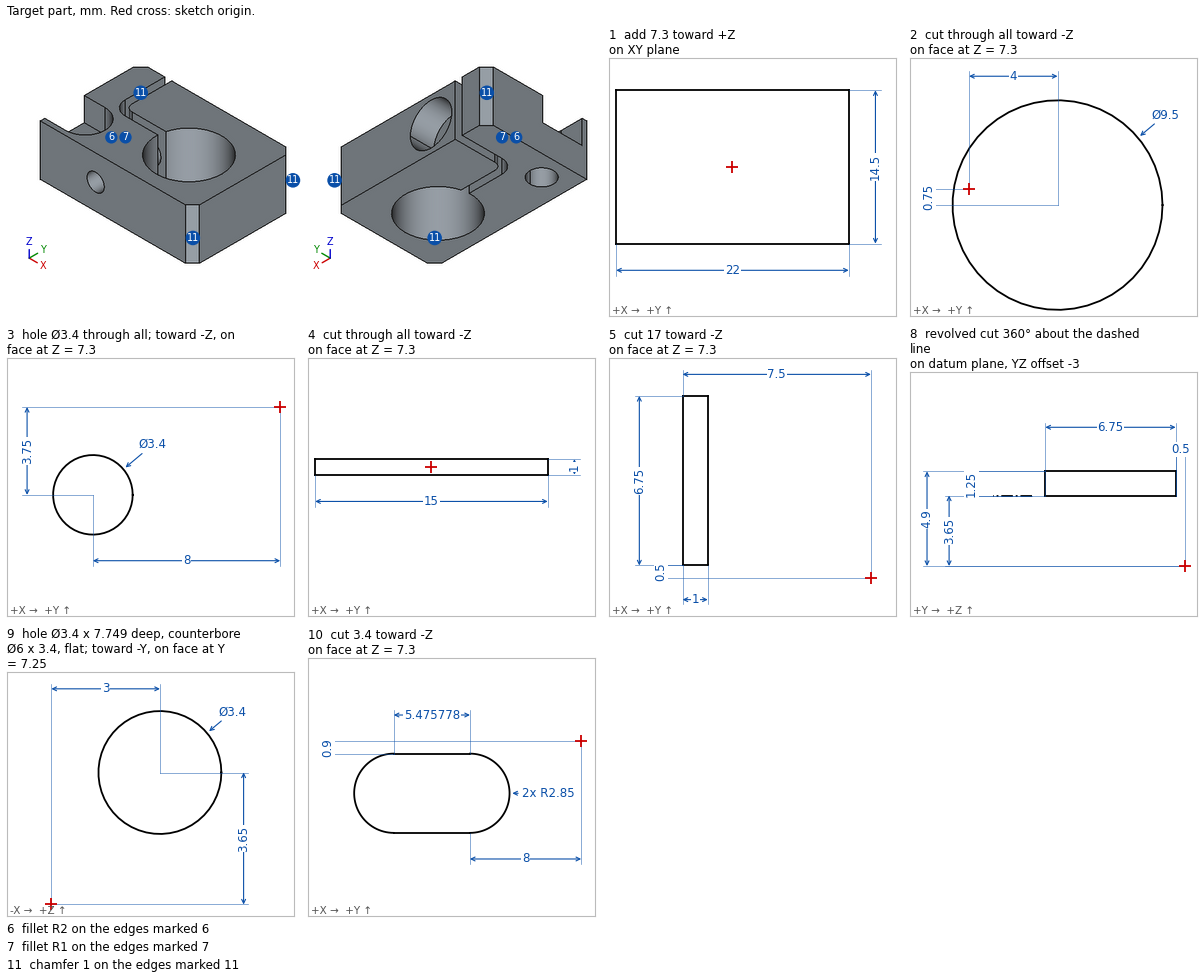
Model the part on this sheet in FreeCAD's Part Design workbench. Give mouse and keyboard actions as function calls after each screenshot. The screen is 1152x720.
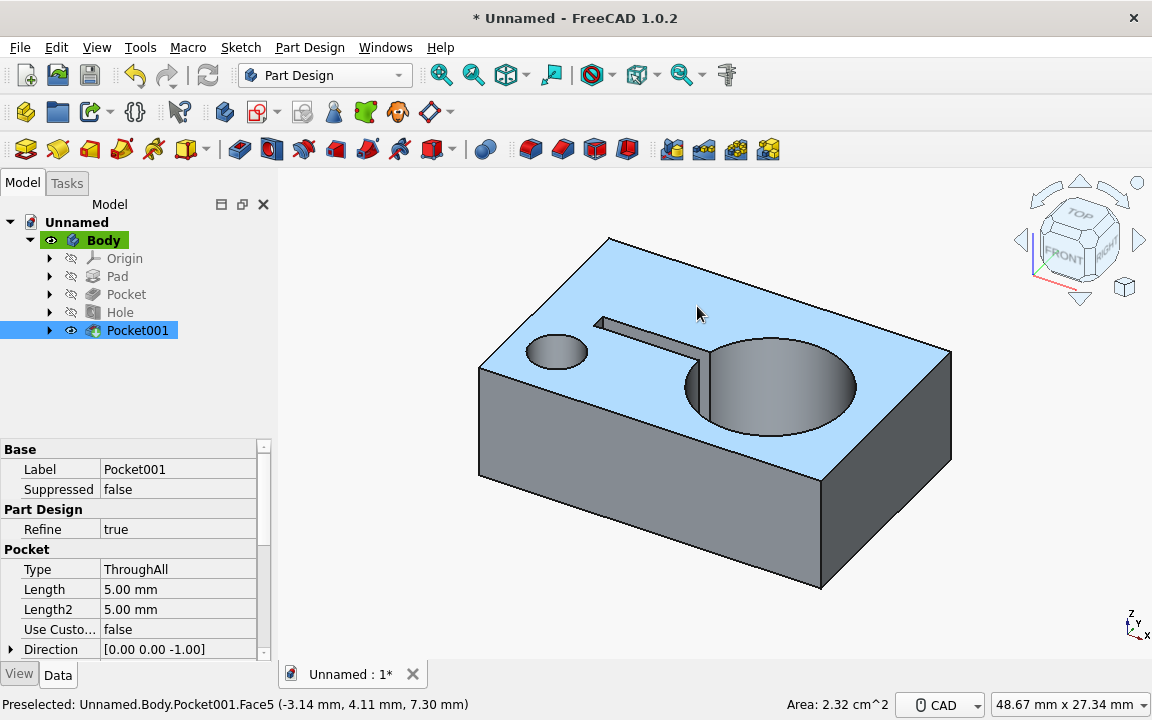
click(258, 112)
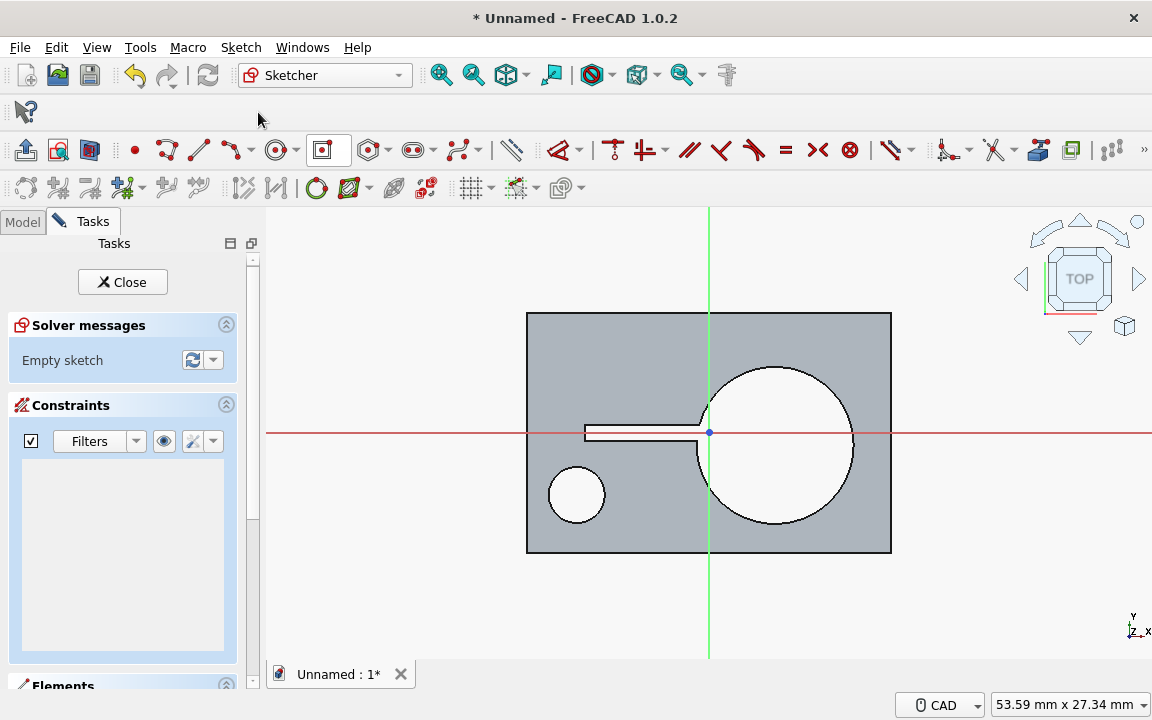
scroll(652, 324, up, 4)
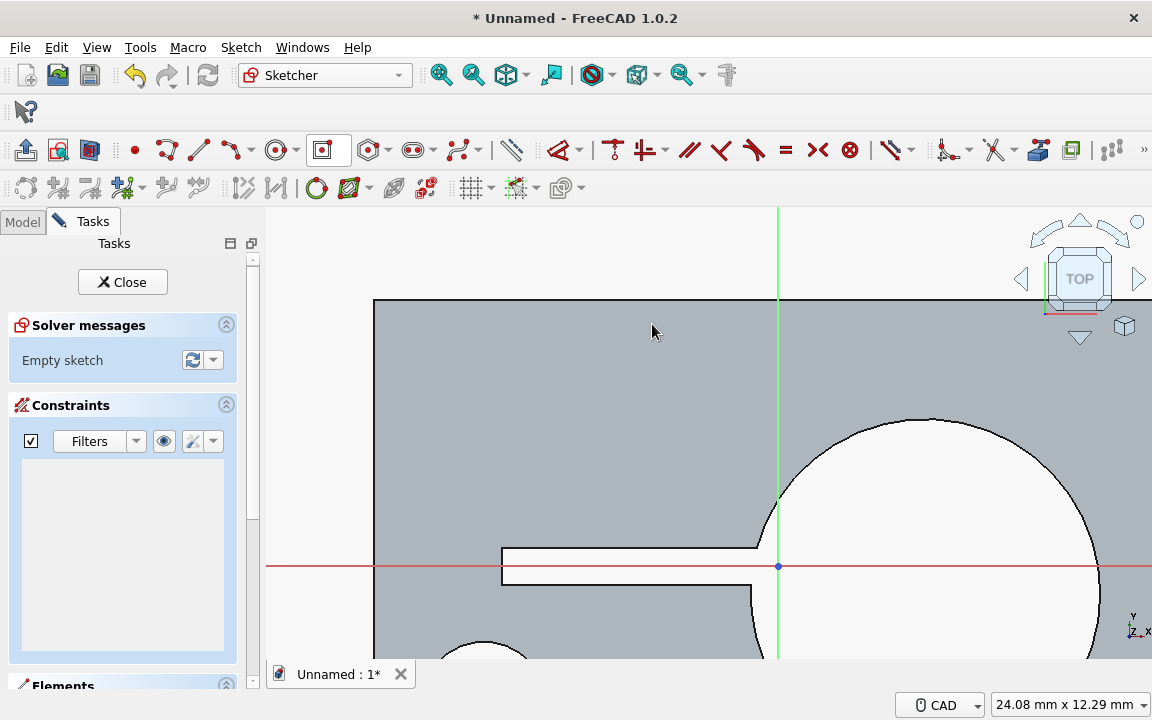
click(346, 150)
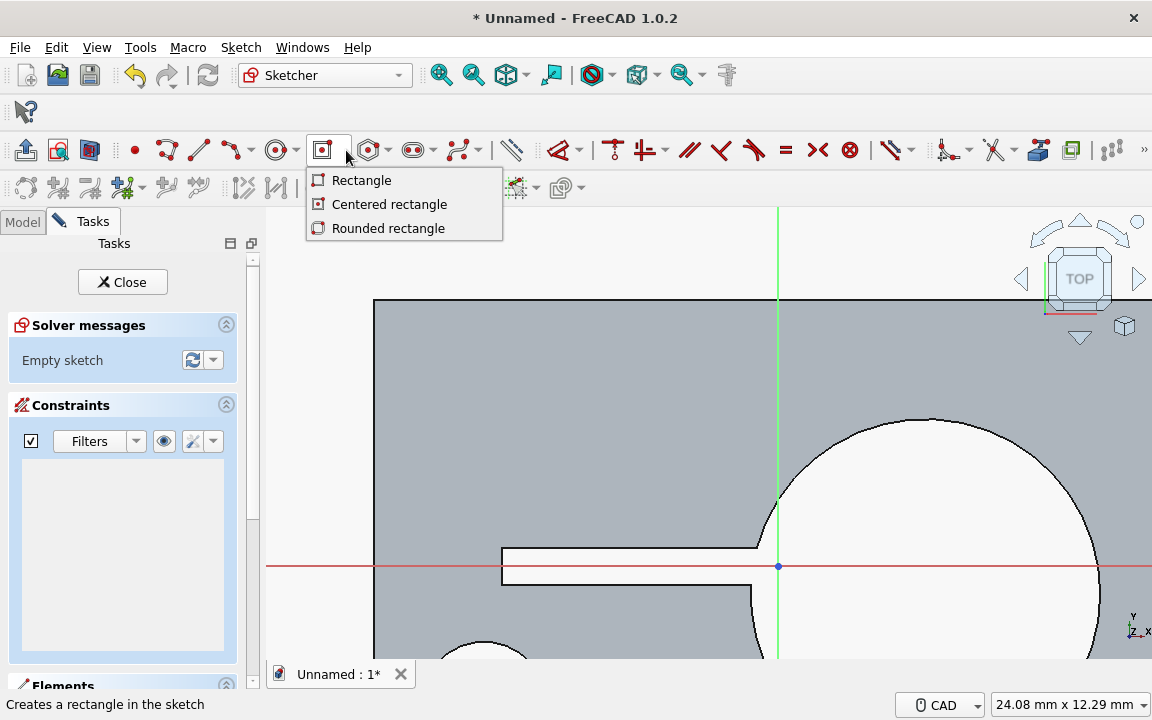
click(404, 180)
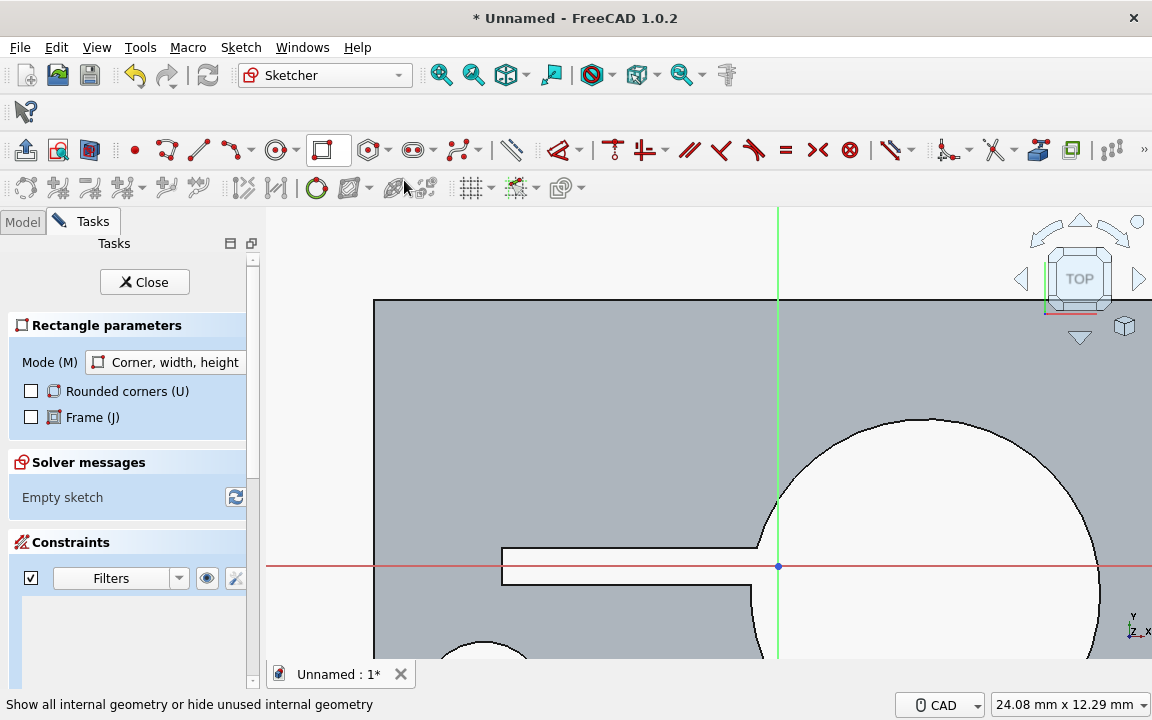
click(502, 300)
click(539, 548)
key(Escape)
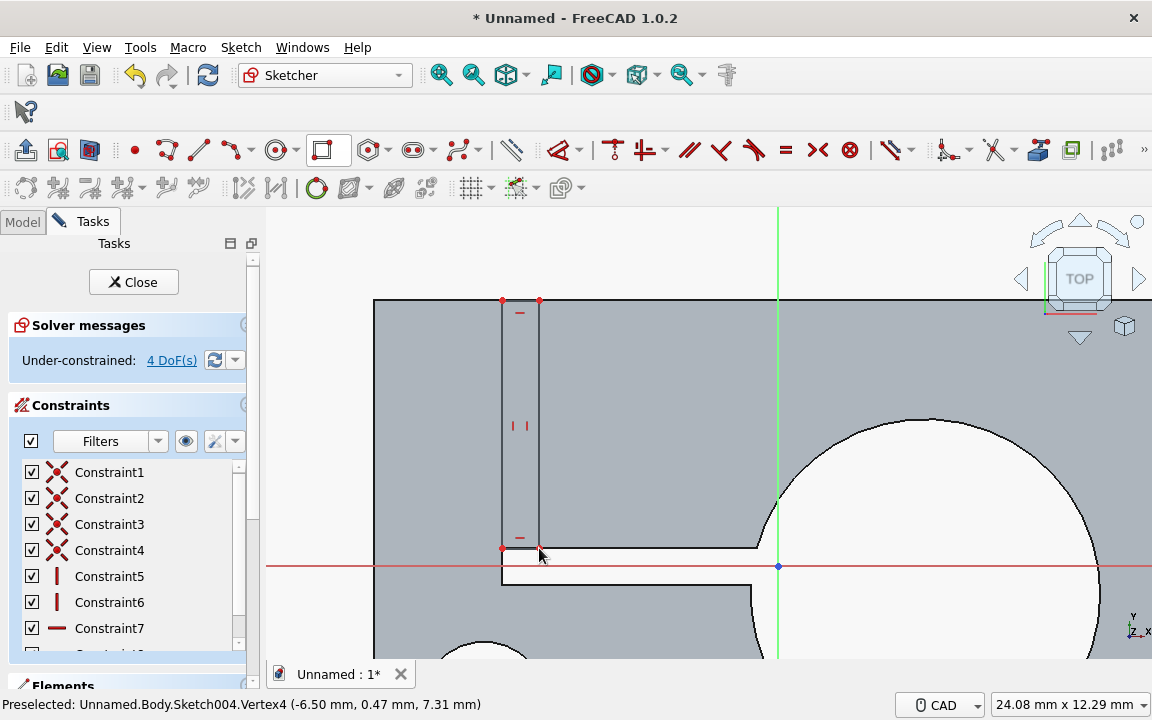
click(558, 150)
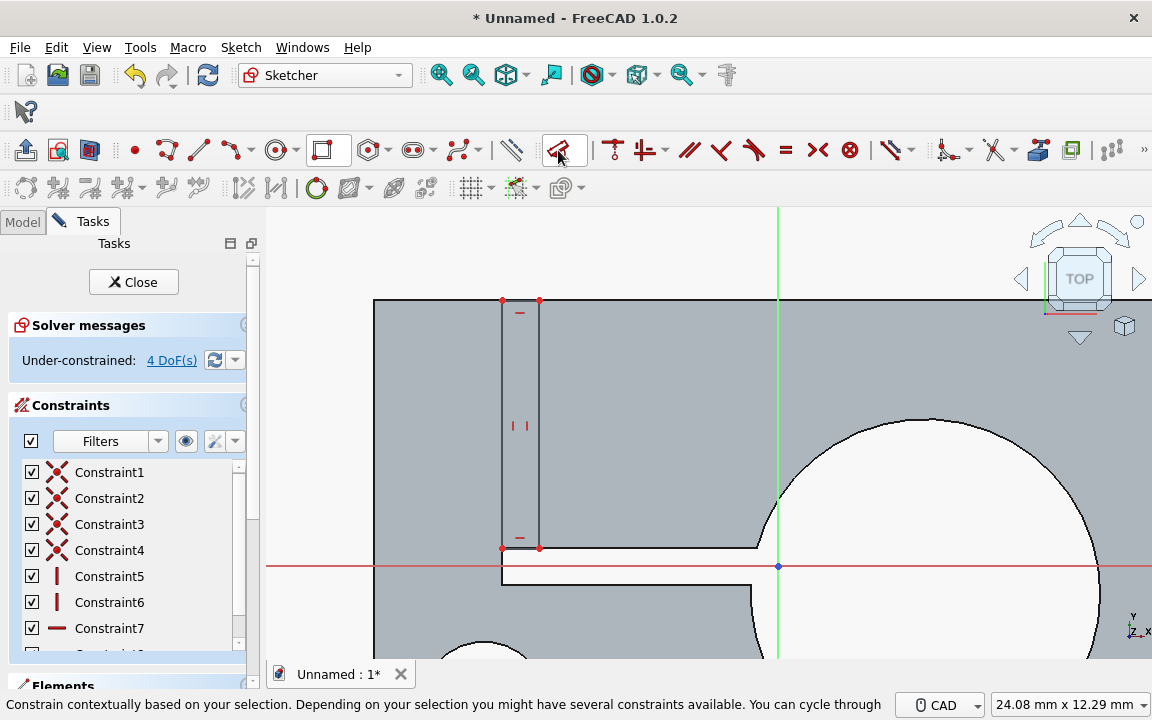
scroll(513, 549, up, 2)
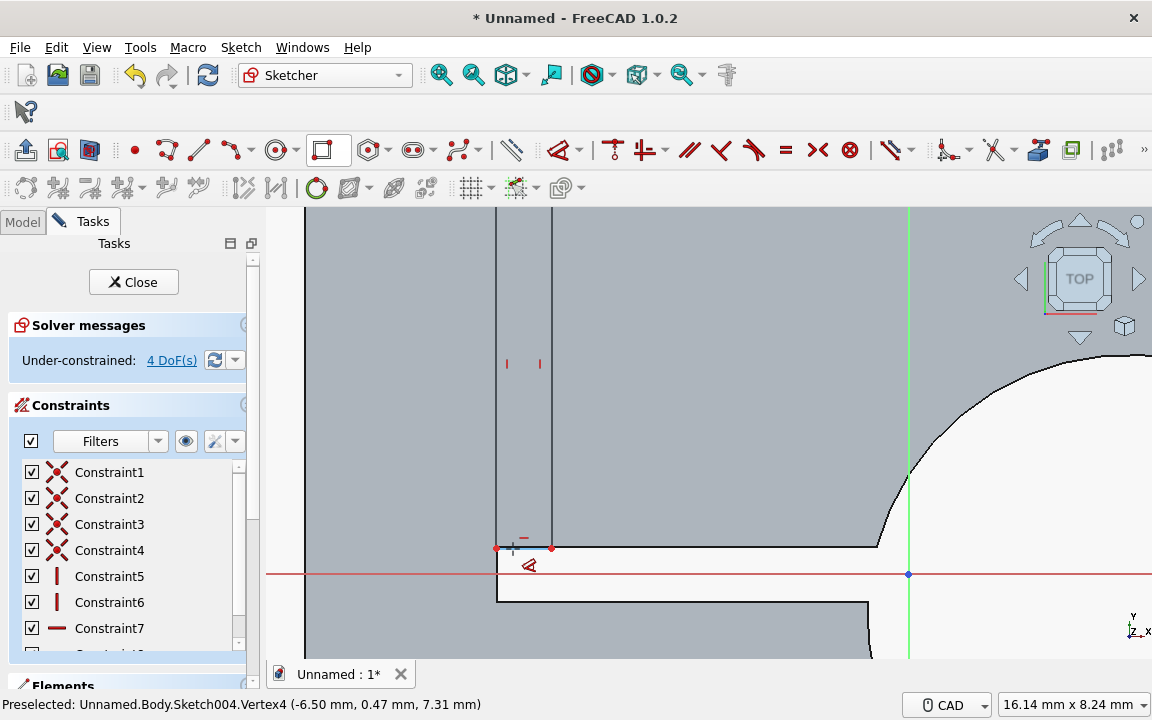
click(513, 549)
click(524, 515)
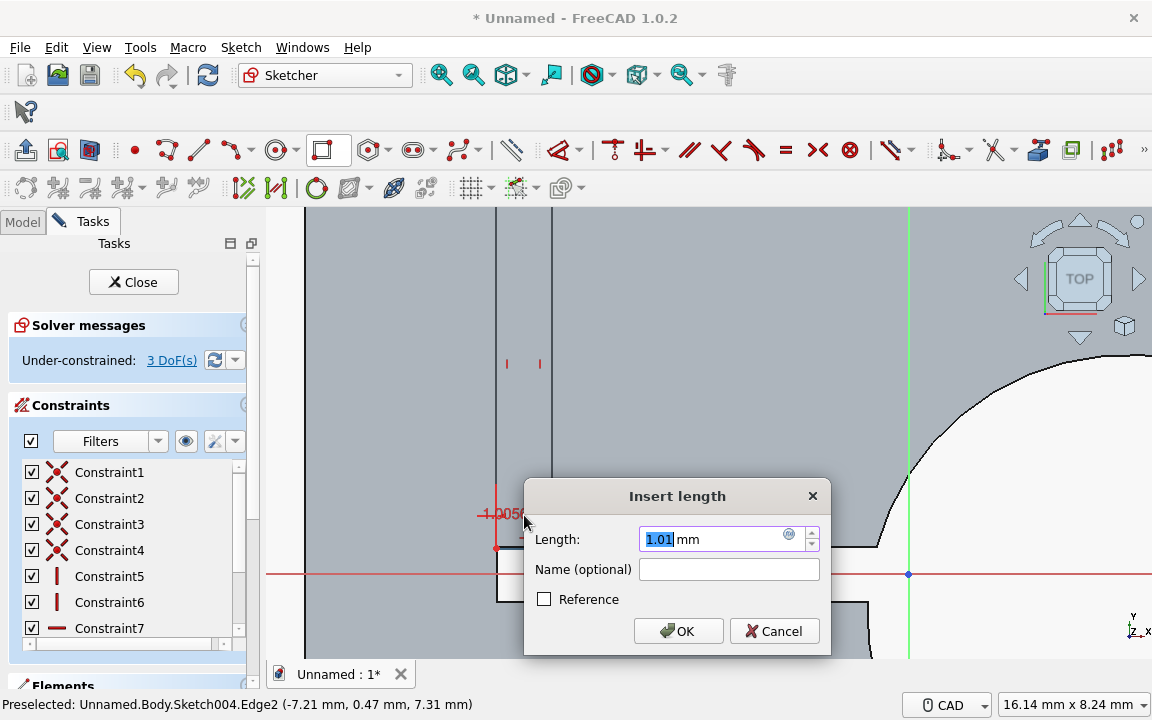
text(1)
key(Return)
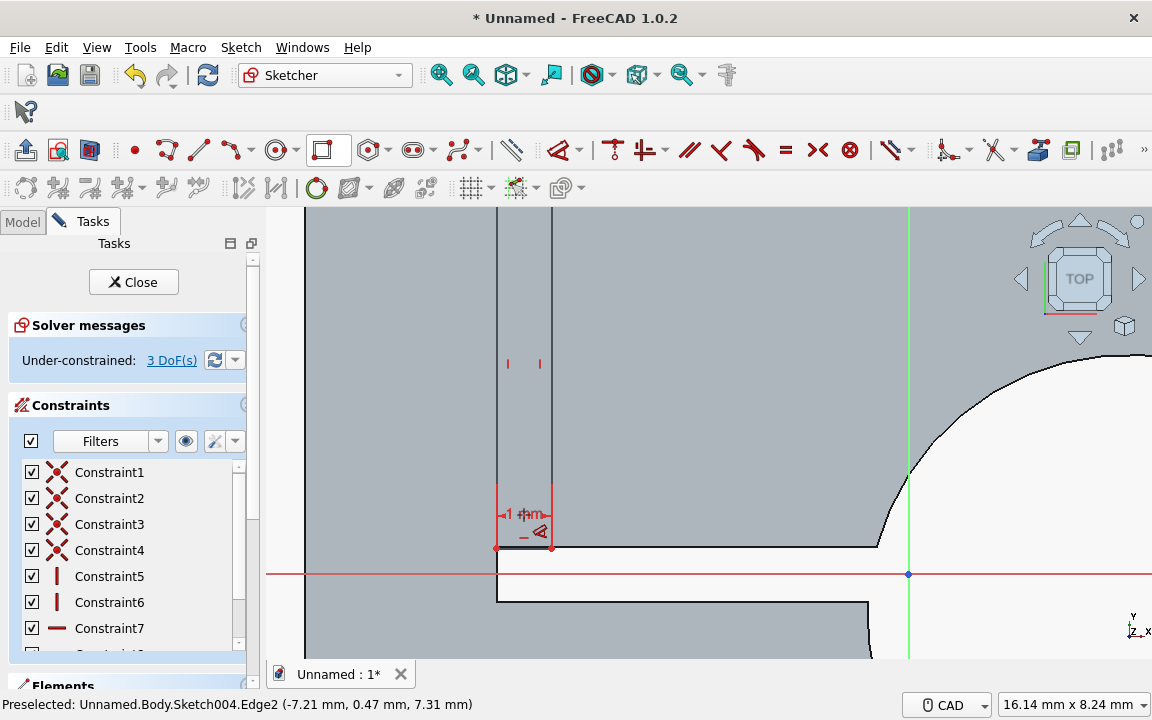
click(497, 290)
click(463, 392)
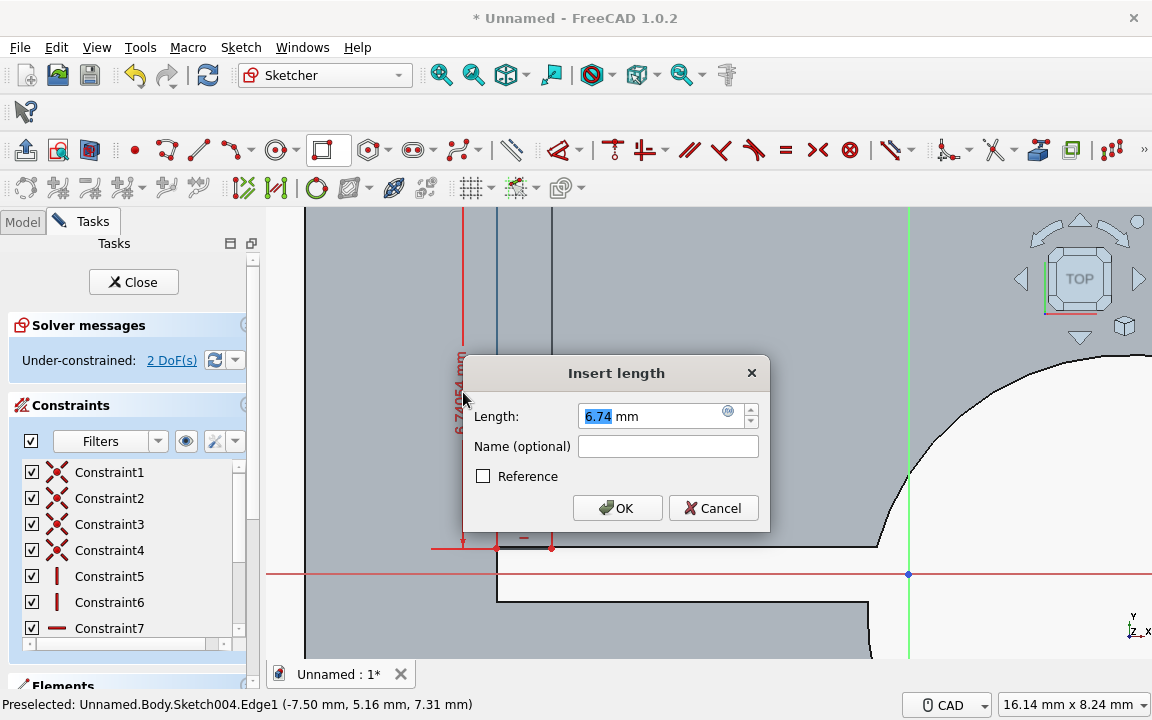
text(6.75)
key(Return)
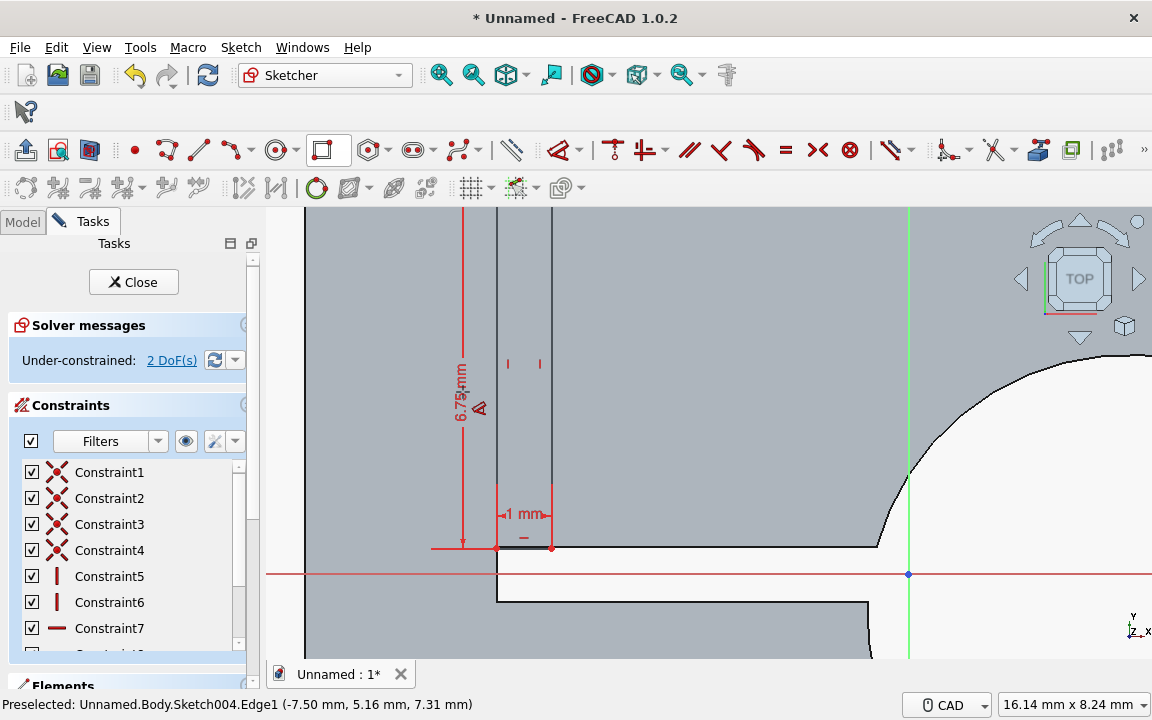
scroll(514, 550, down, 2)